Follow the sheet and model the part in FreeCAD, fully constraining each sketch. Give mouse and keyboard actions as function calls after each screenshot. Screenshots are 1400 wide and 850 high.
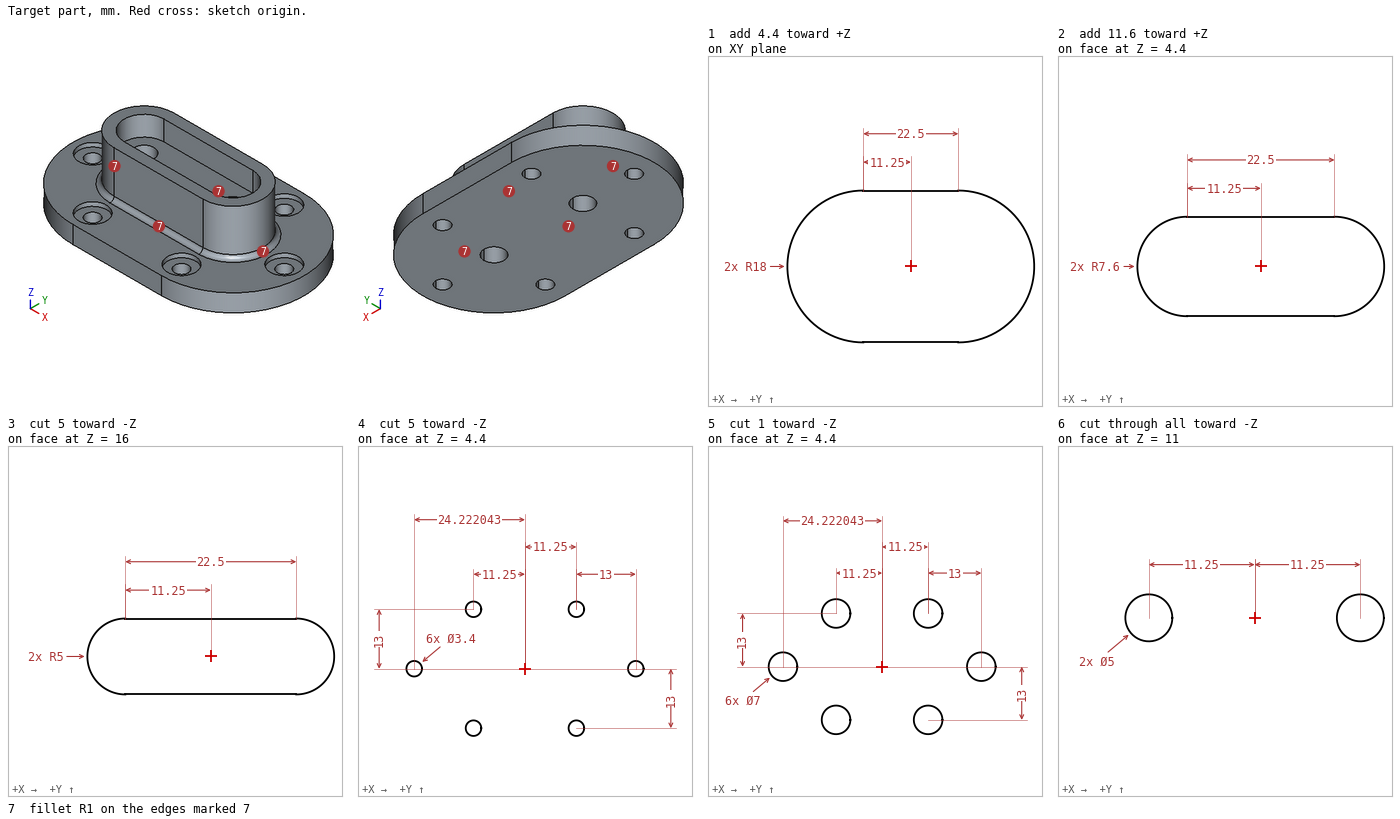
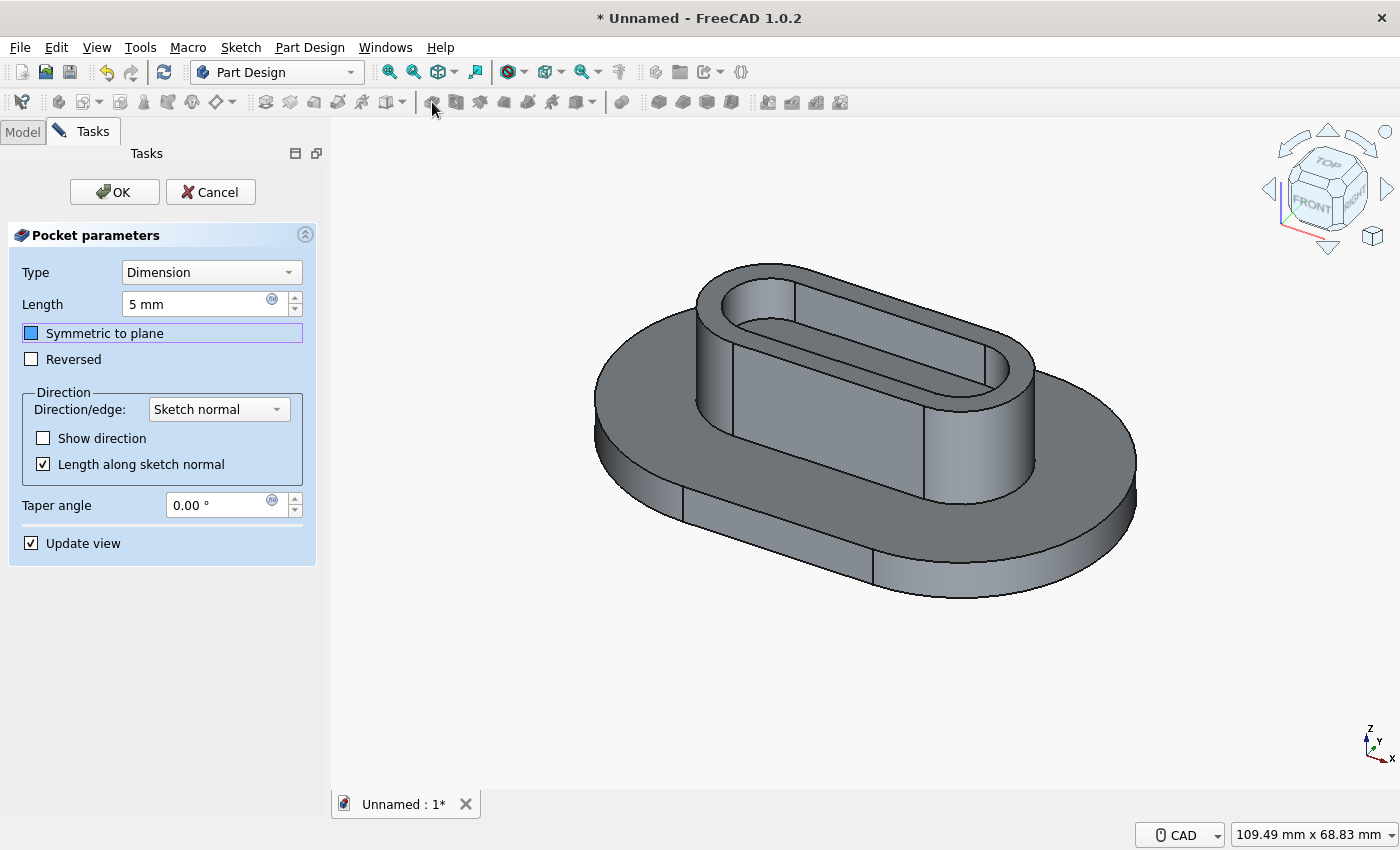
click(115, 192)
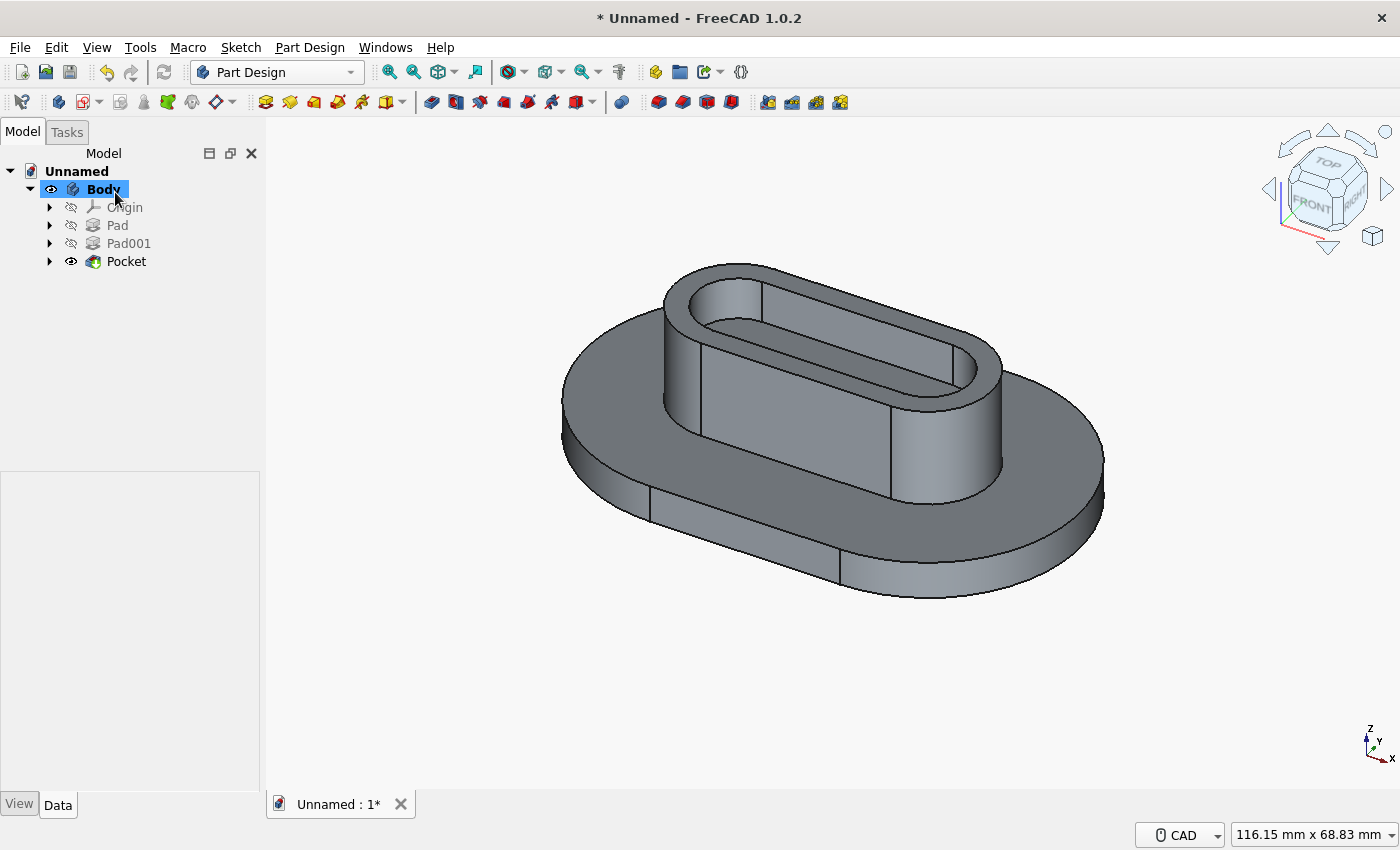
click(1045, 500)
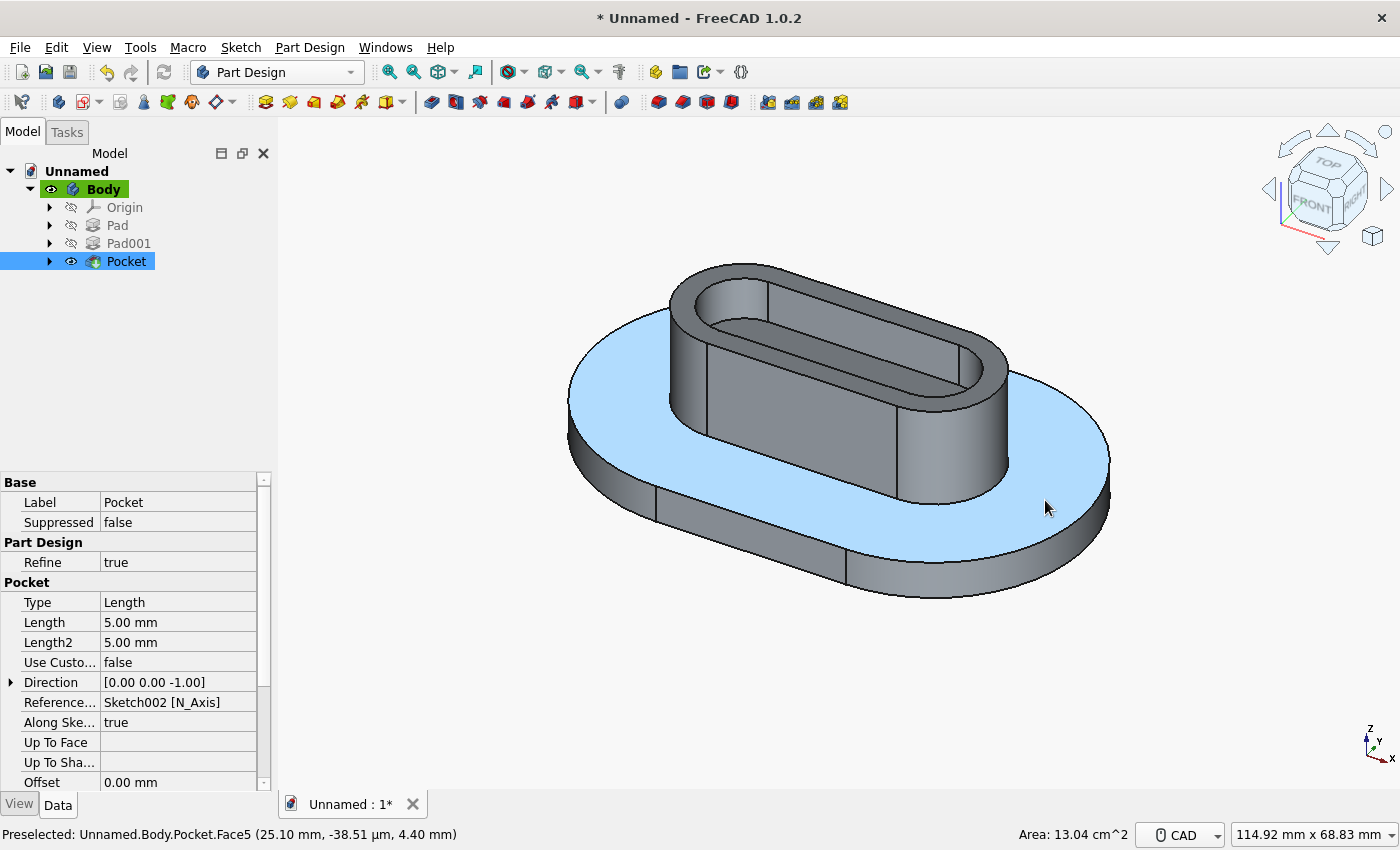
click(84, 102)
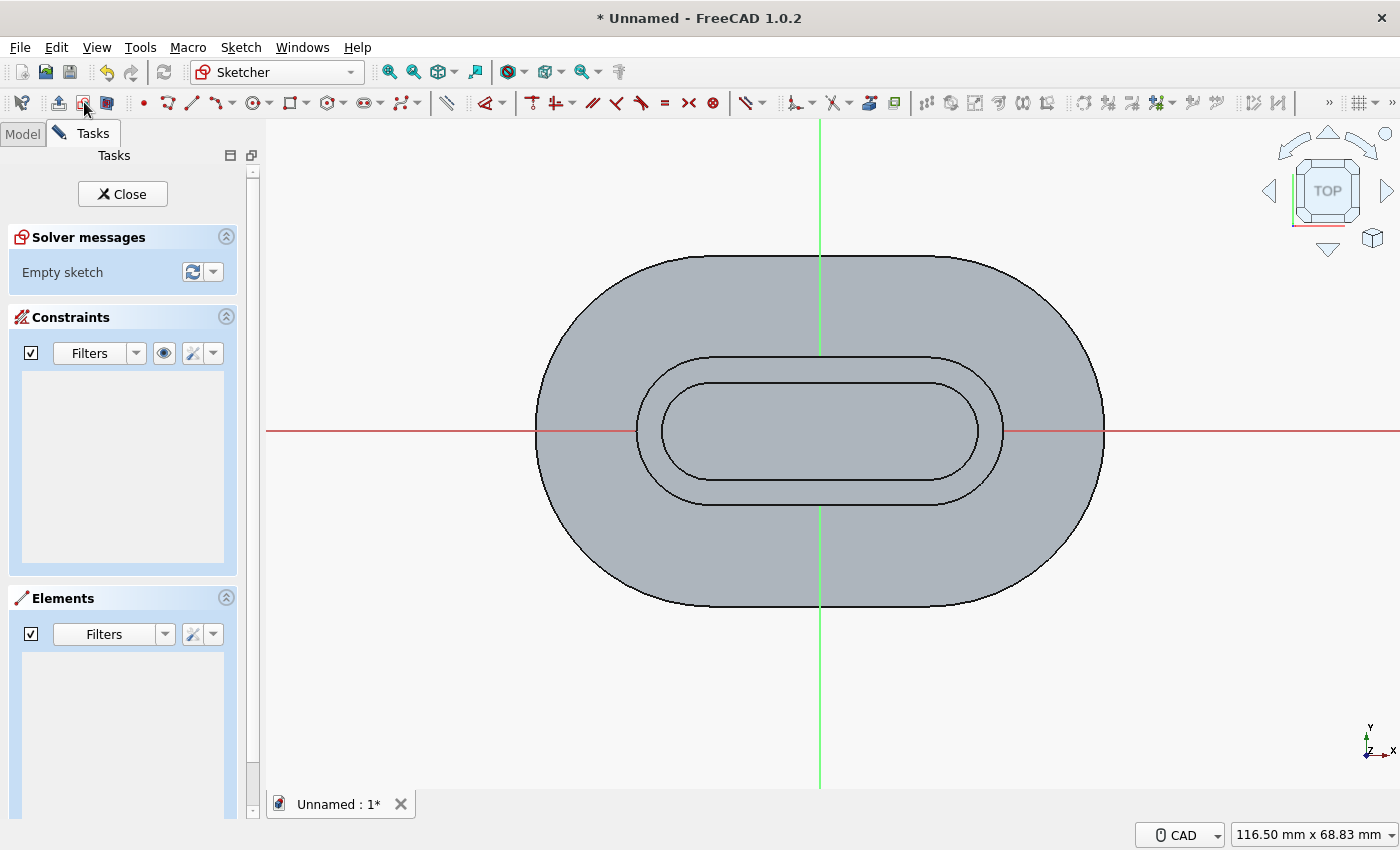
click(108, 104)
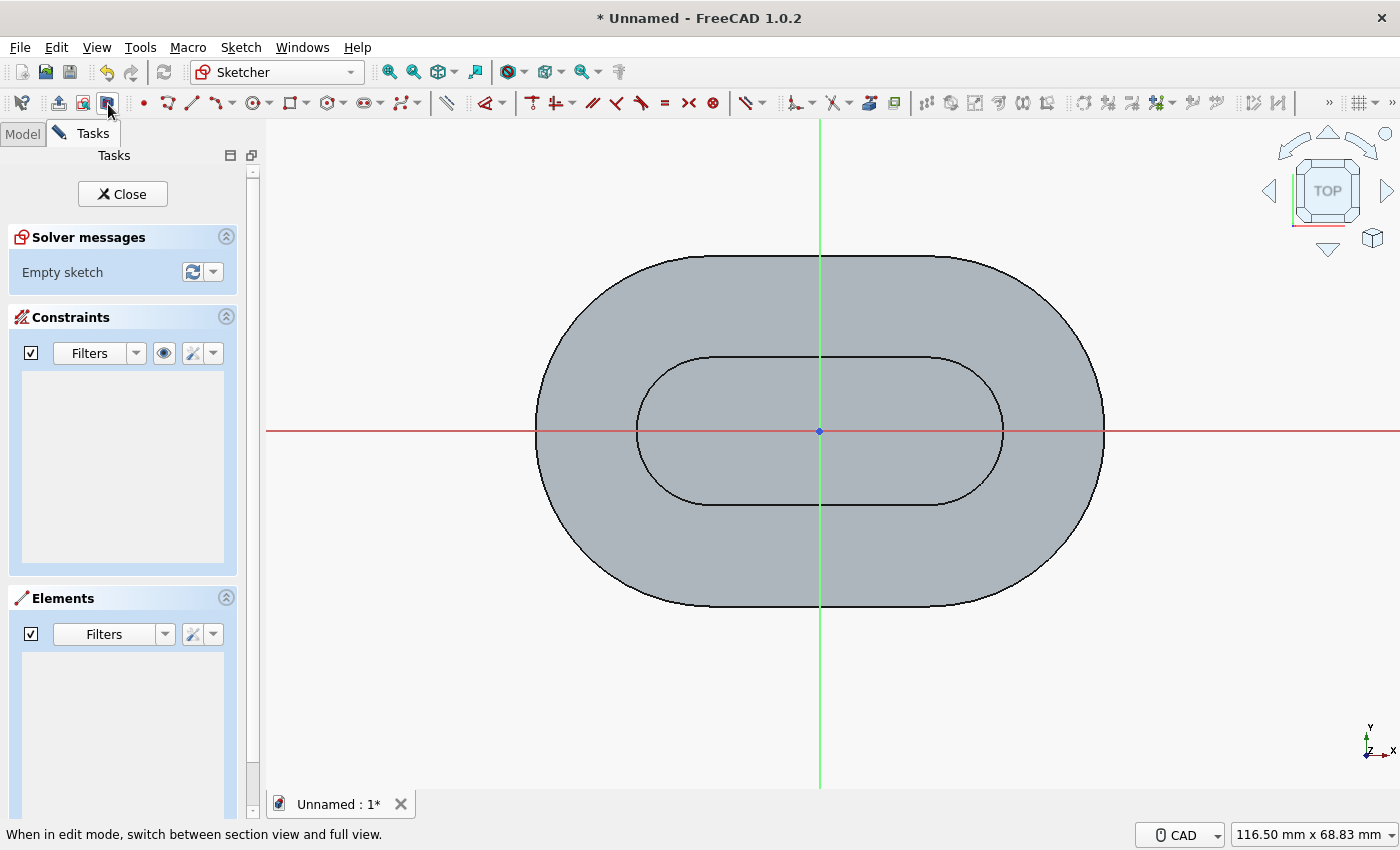
click(254, 104)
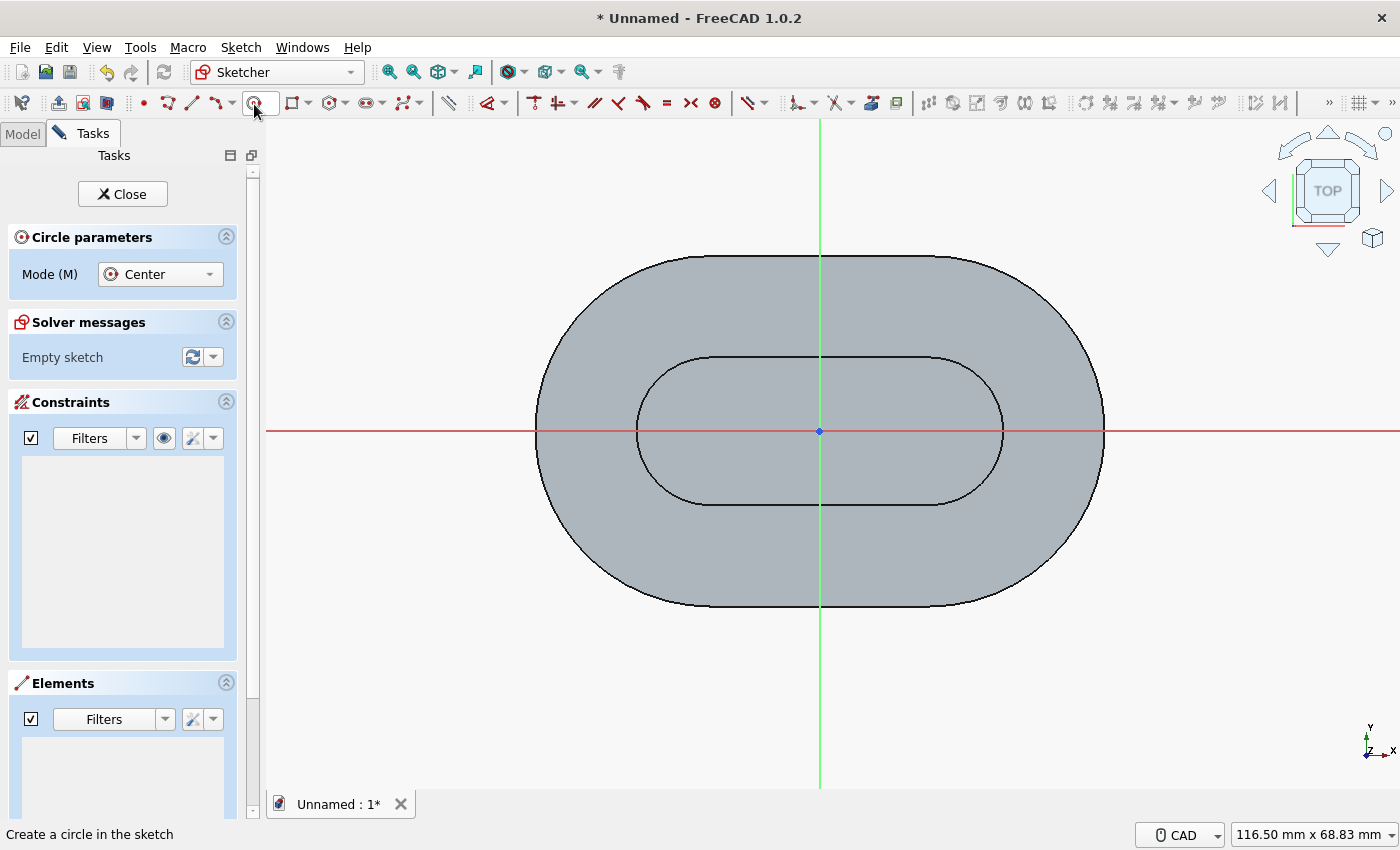
scroll(584, 431, up, 2)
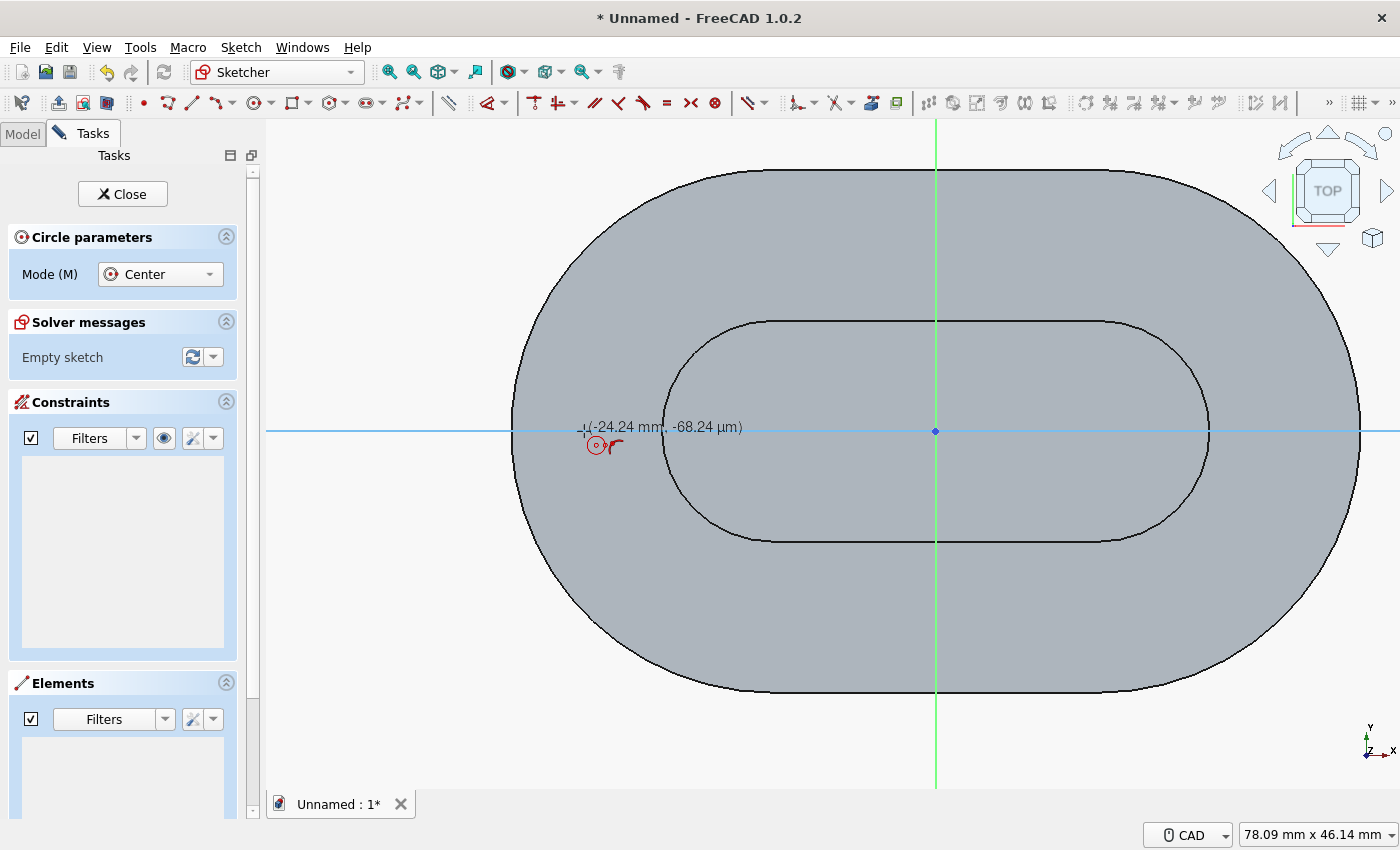
click(584, 431)
move(602, 414)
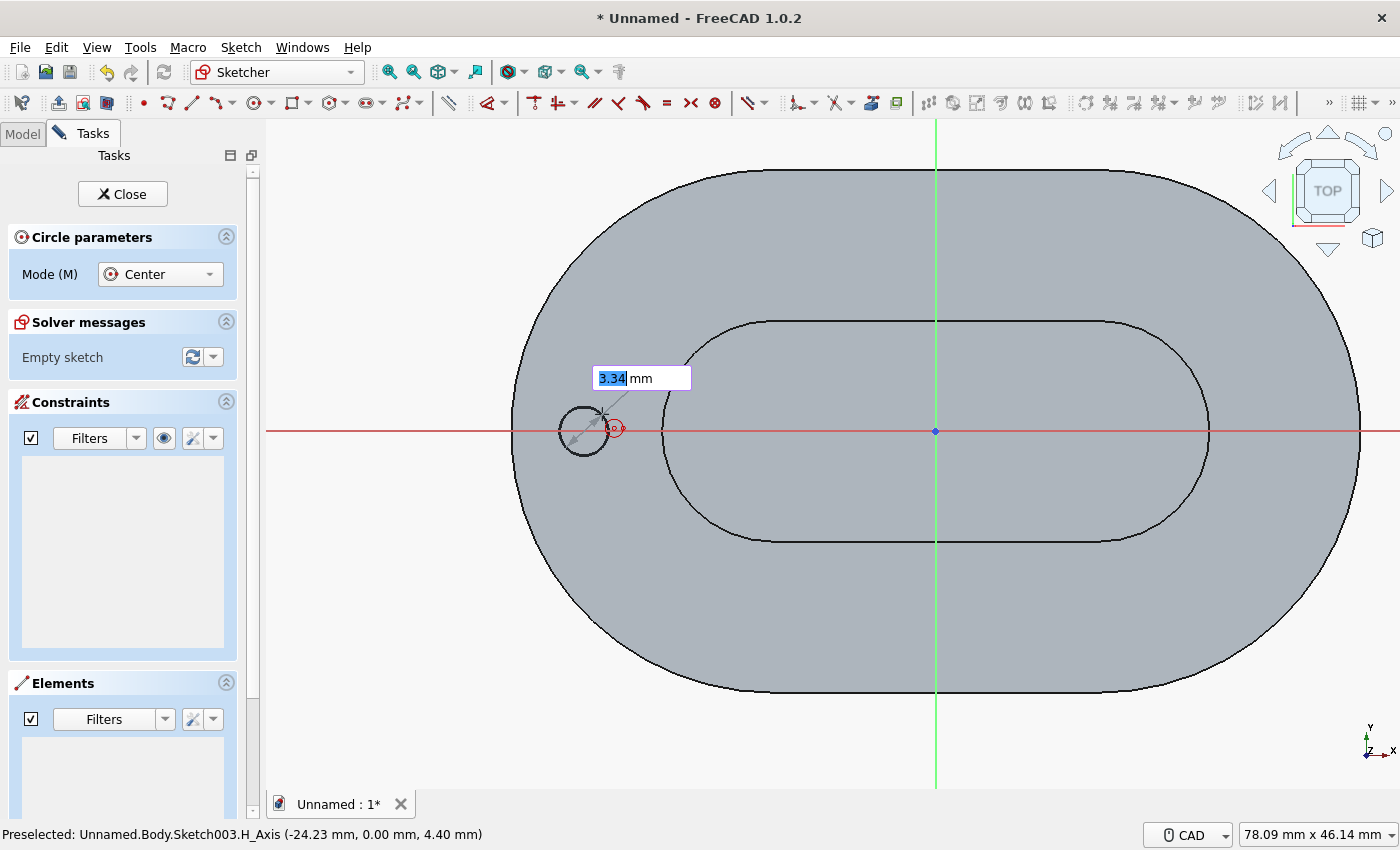
text(3.4)
key(Return)